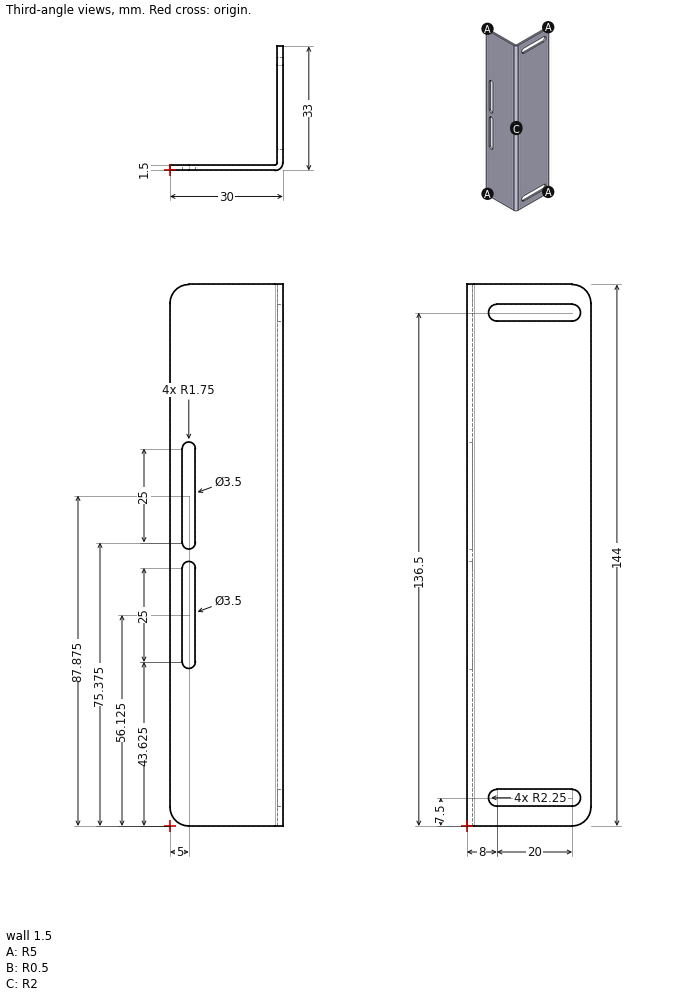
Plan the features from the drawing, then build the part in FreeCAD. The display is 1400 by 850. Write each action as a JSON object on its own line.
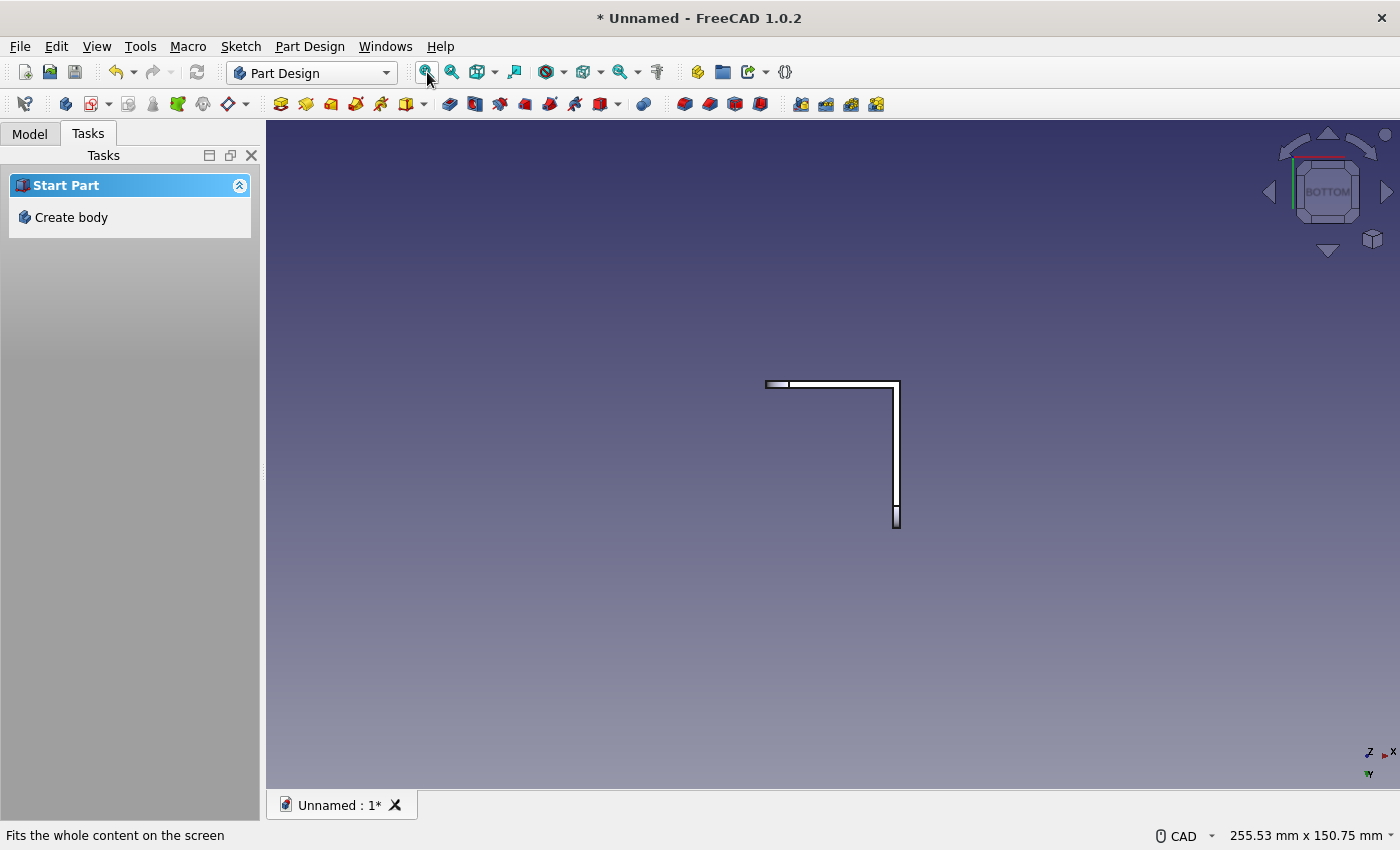
{"action": "key", "text": "4"}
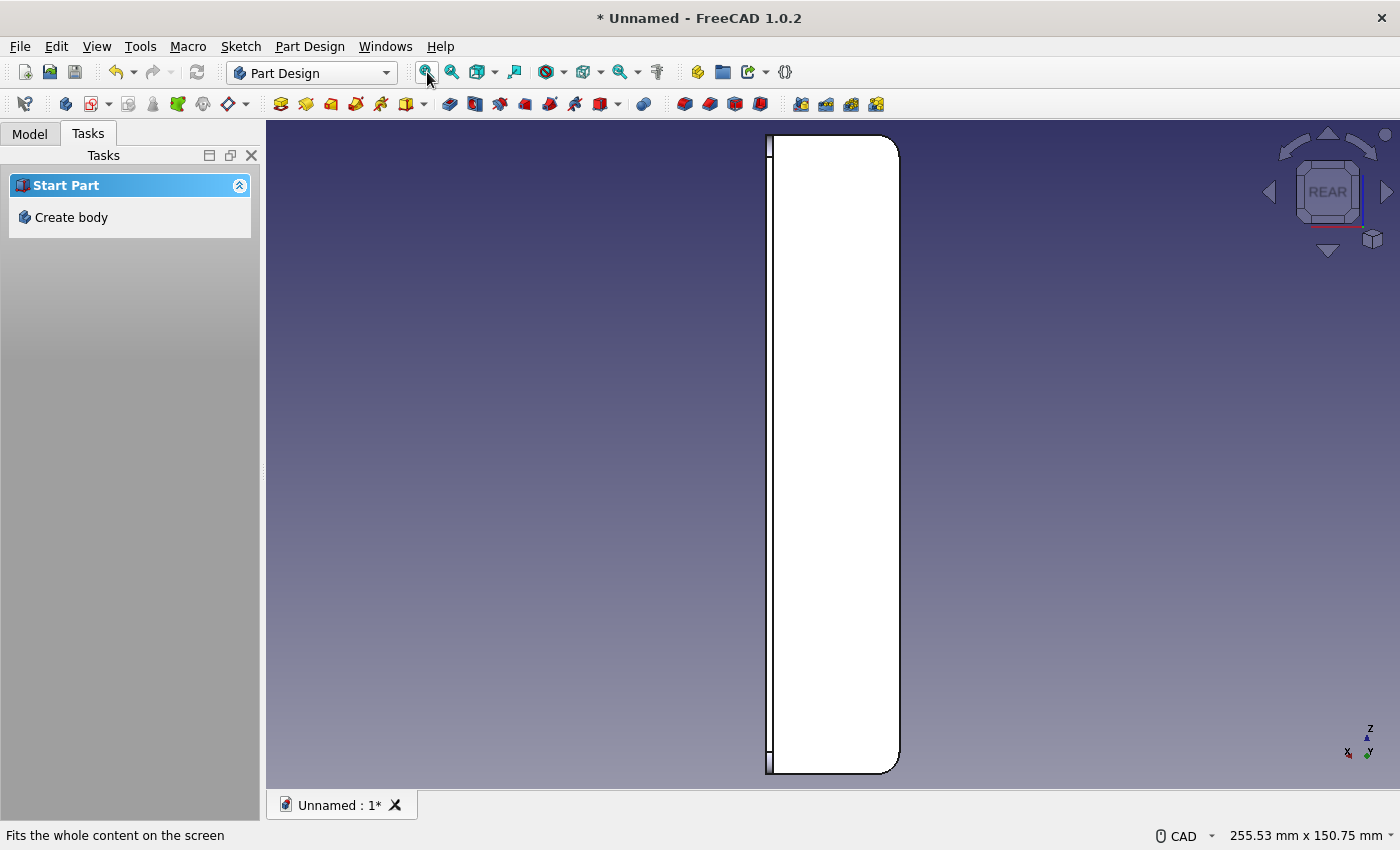
{"action": "key", "text": "6"}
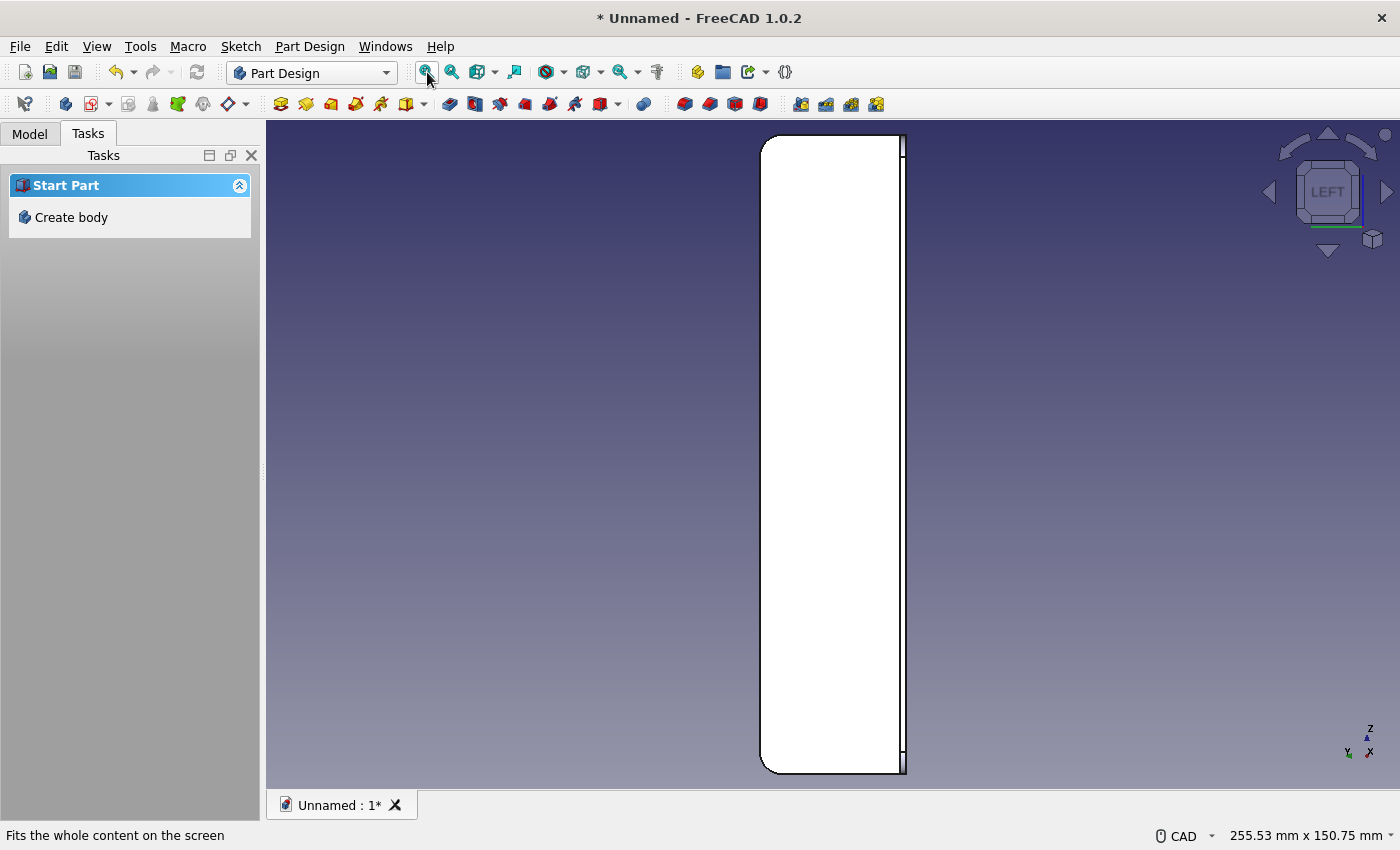
{"action": "key", "text": "v 3"}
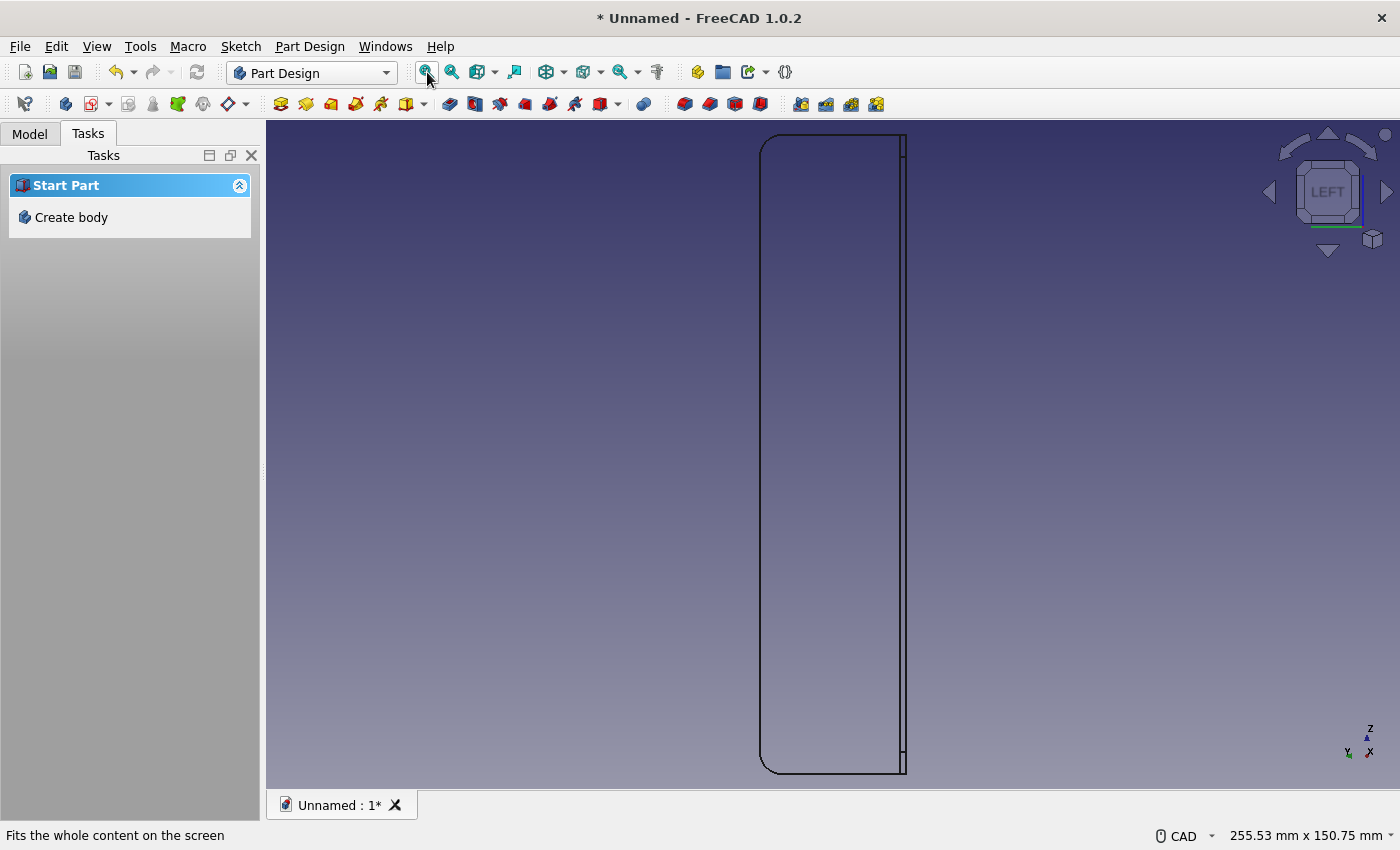
{"action": "key", "text": "0"}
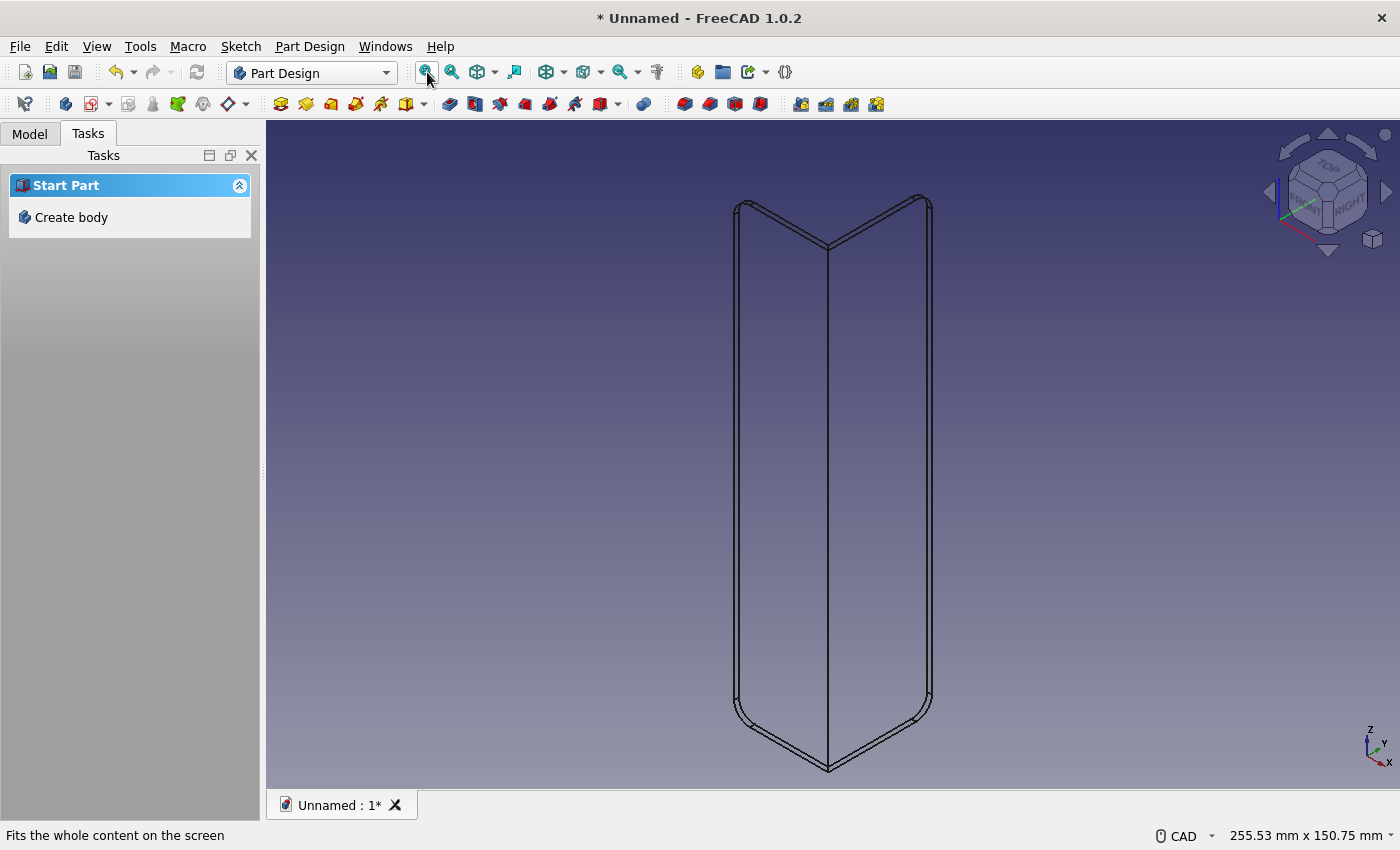
{"action": "key", "text": "2"}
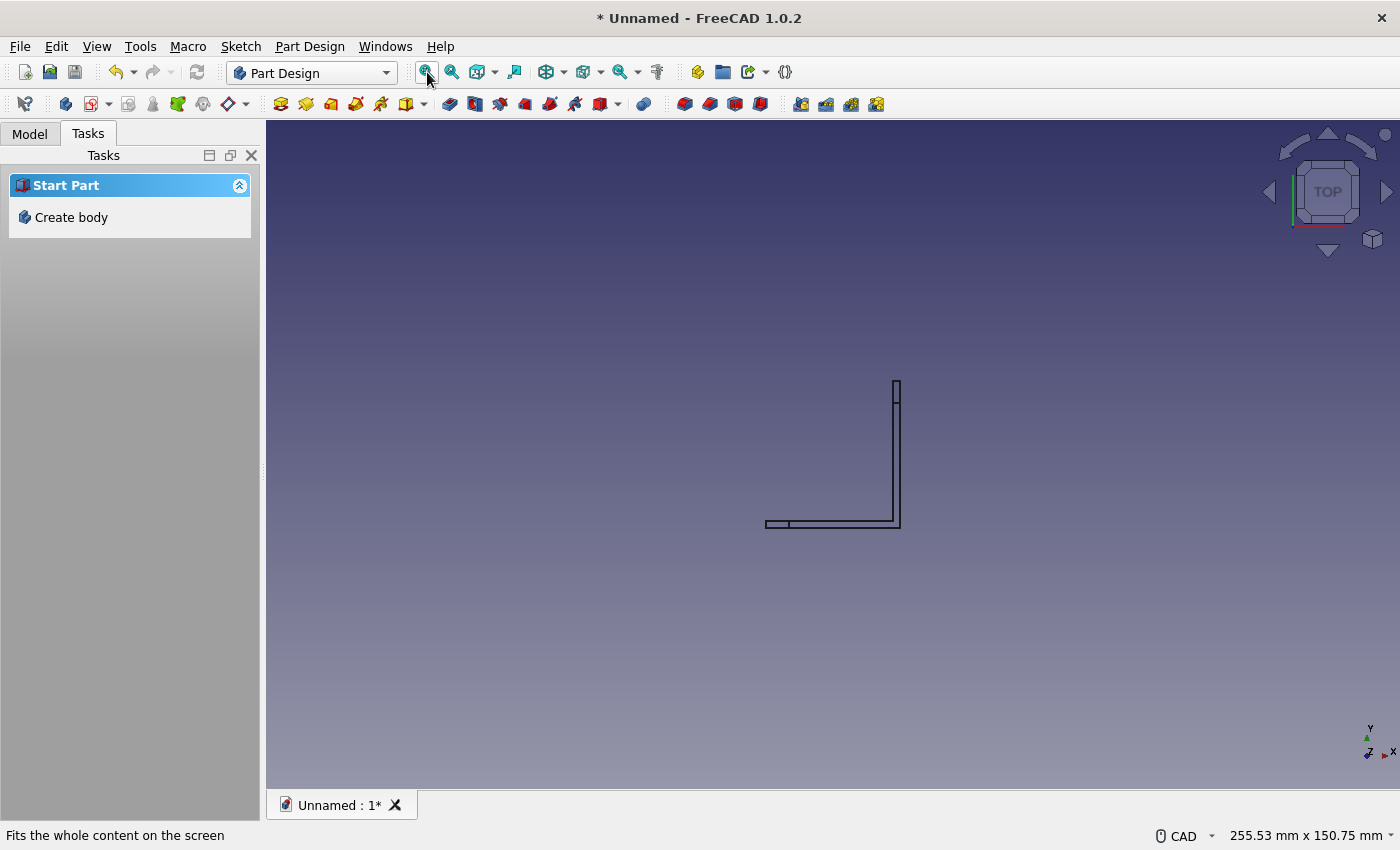
{"action": "left_click", "coordinate": [427, 72]}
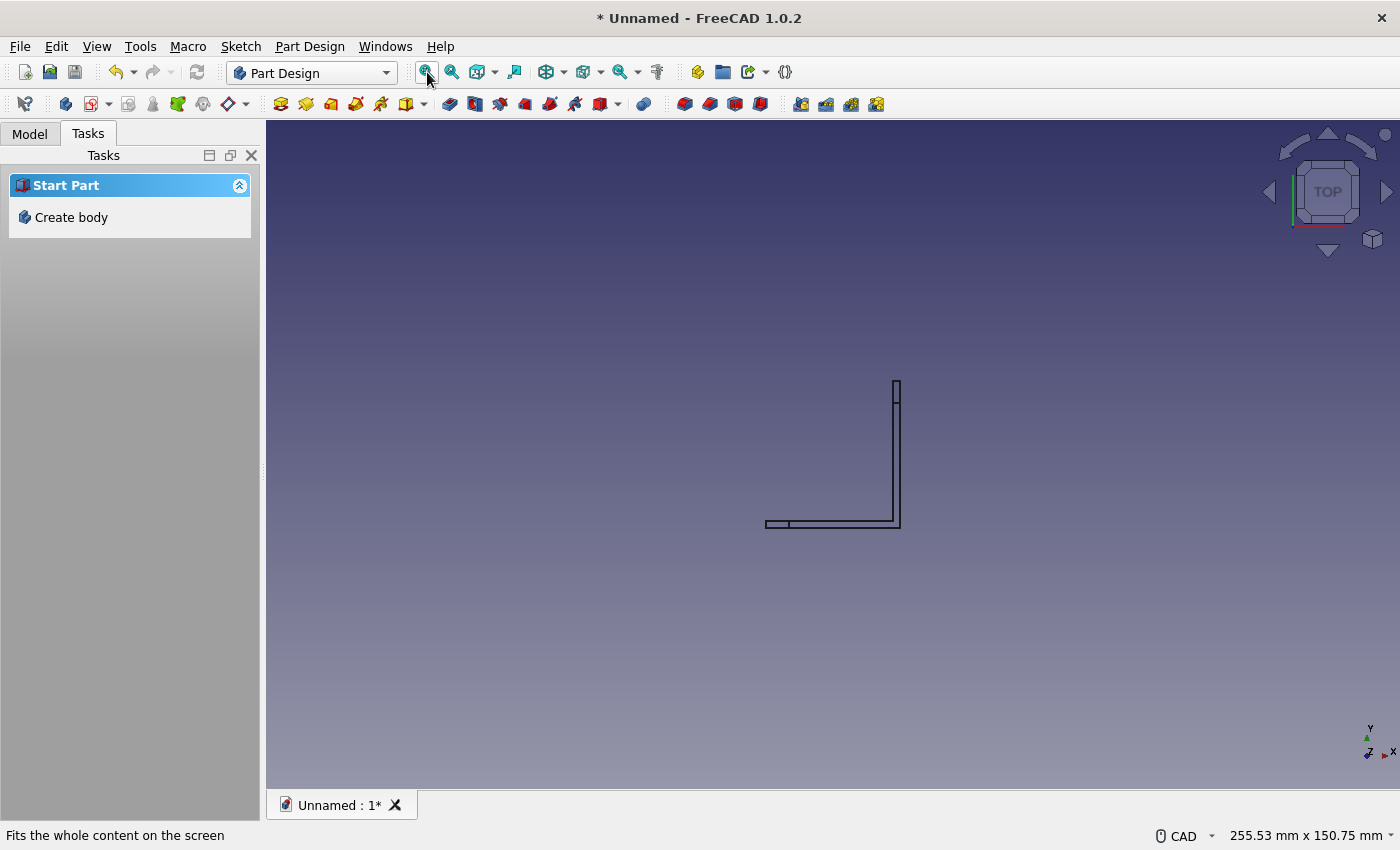
{"action": "key", "text": "1"}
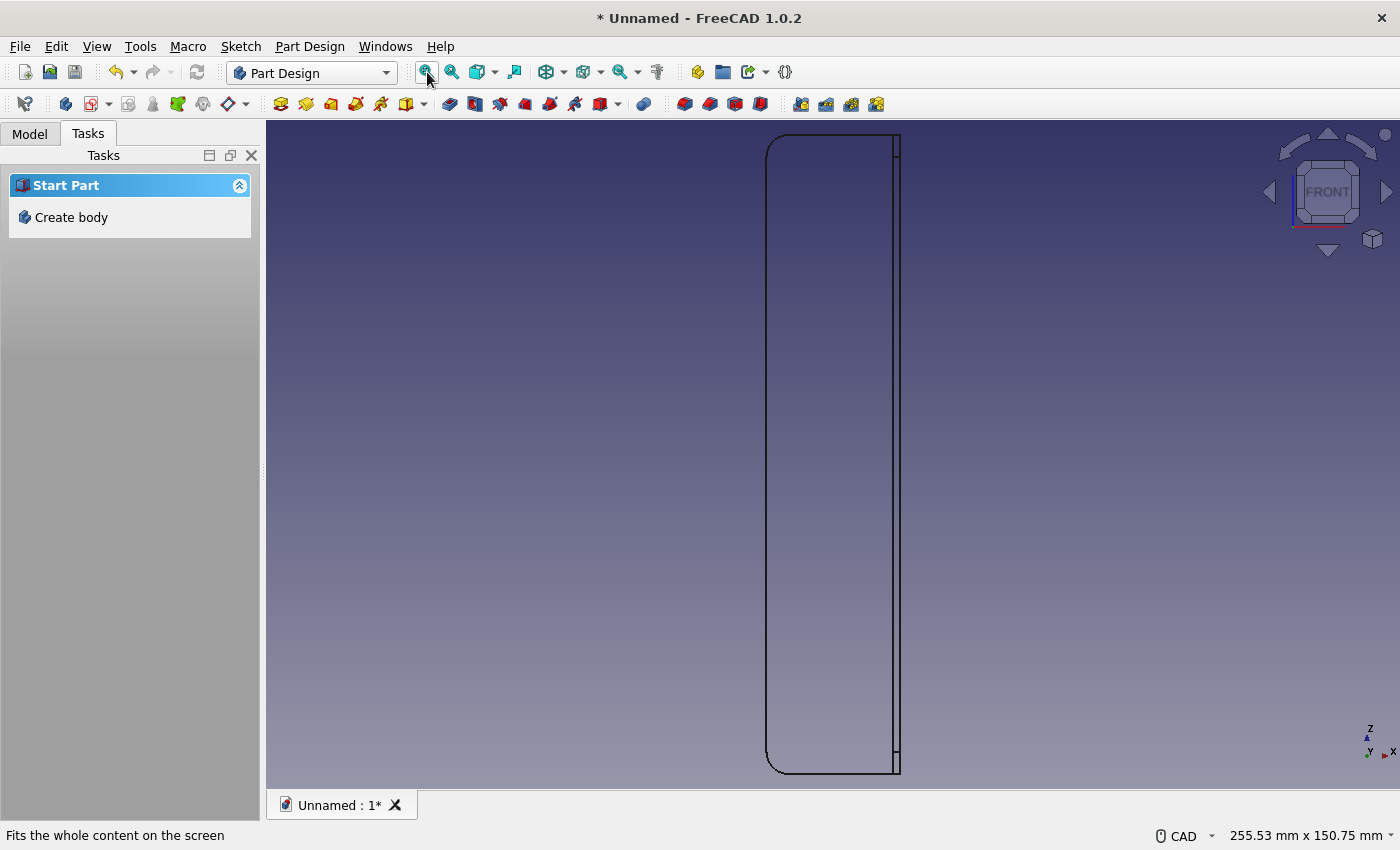
{"action": "left_click", "coordinate": [893, 453]}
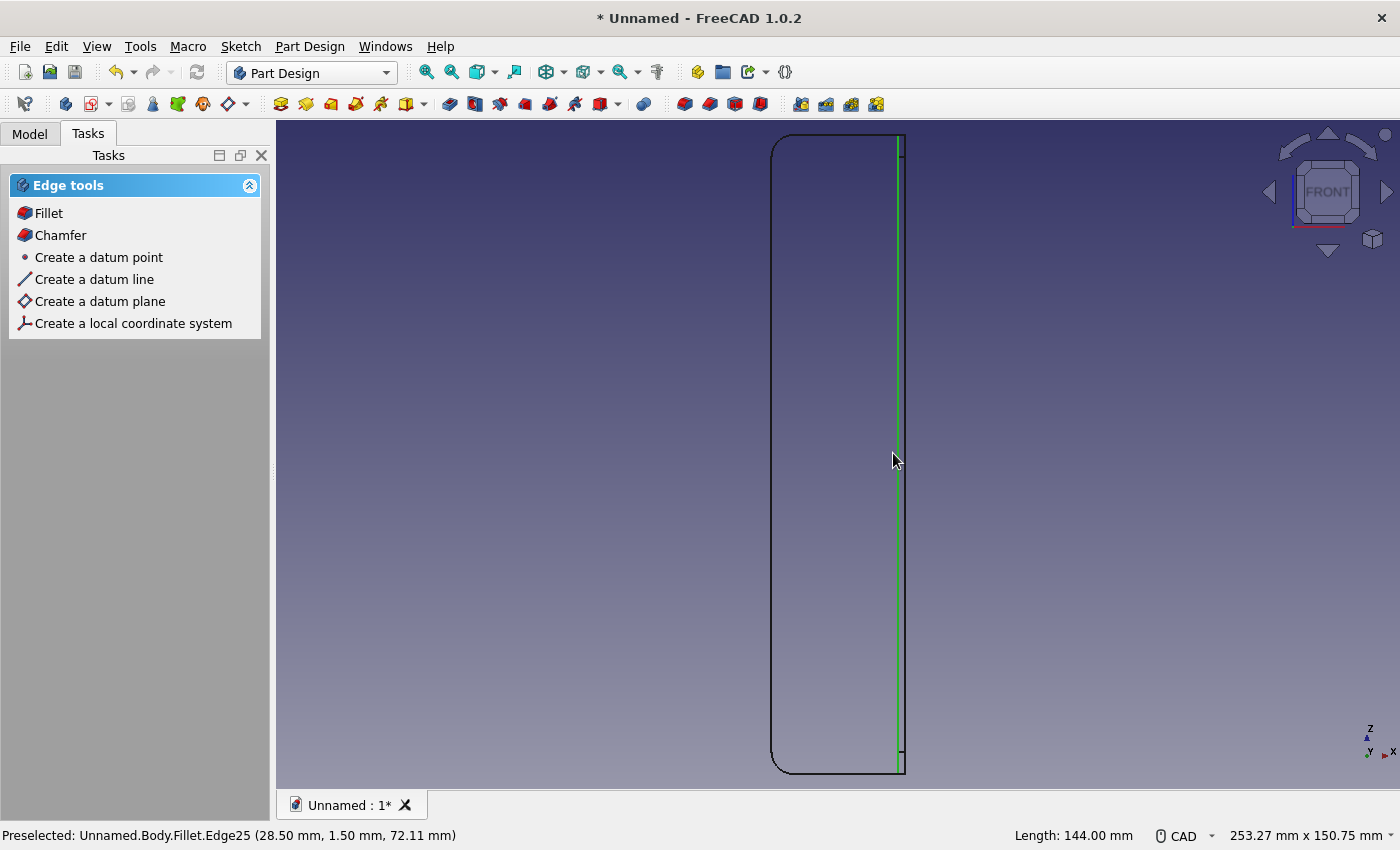
{"action": "key", "text": "v 1"}